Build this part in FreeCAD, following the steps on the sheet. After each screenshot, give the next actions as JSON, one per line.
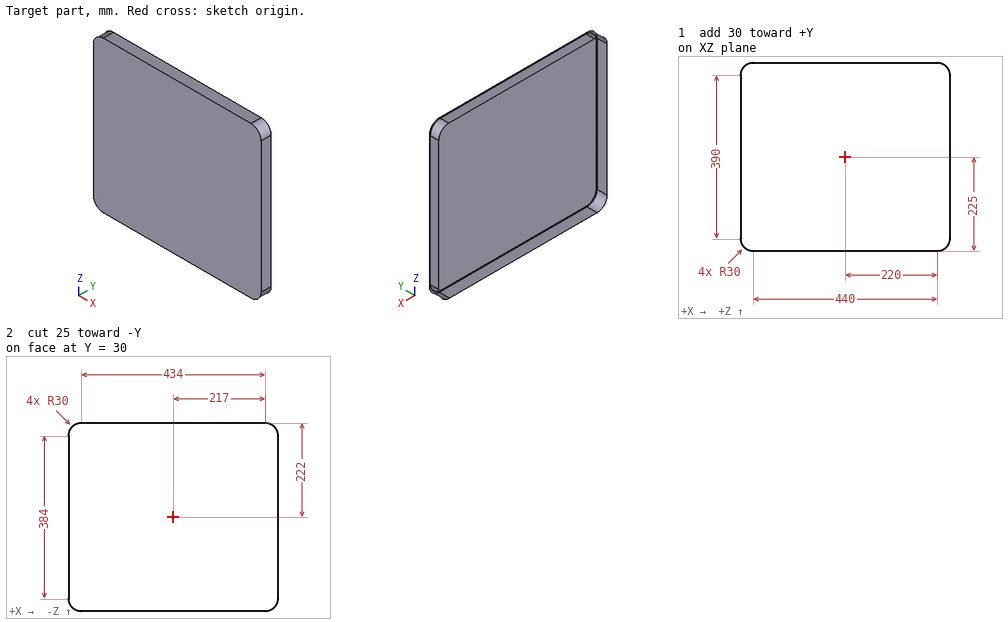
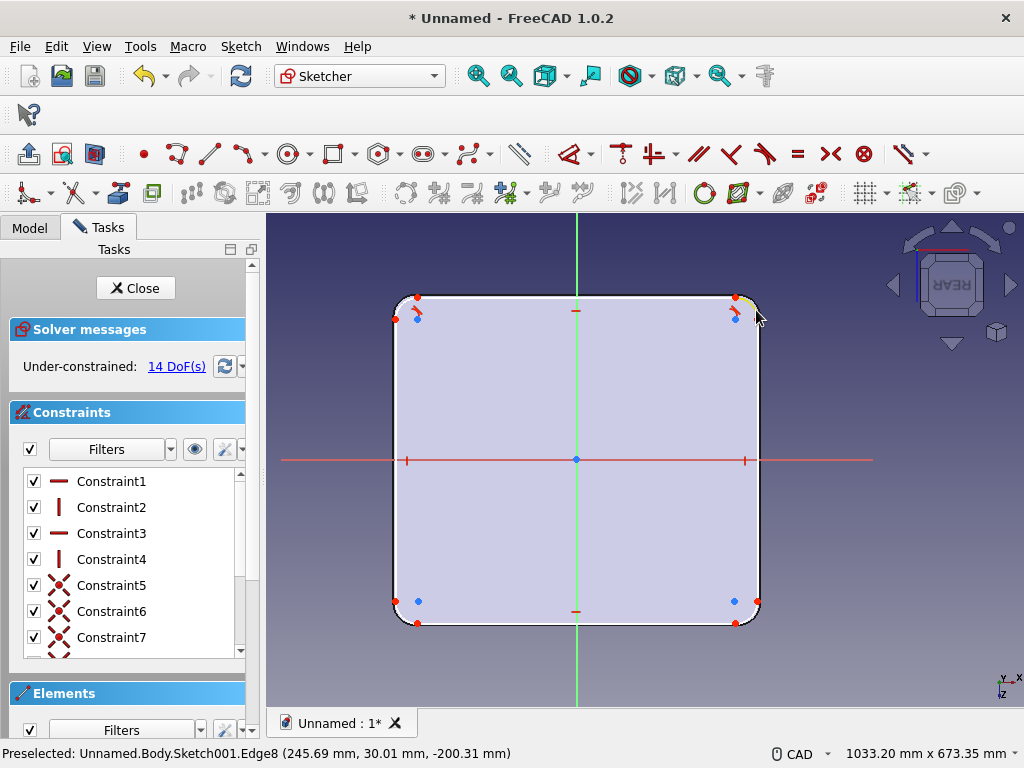
{"action": "left_click", "coordinate": [396, 405]}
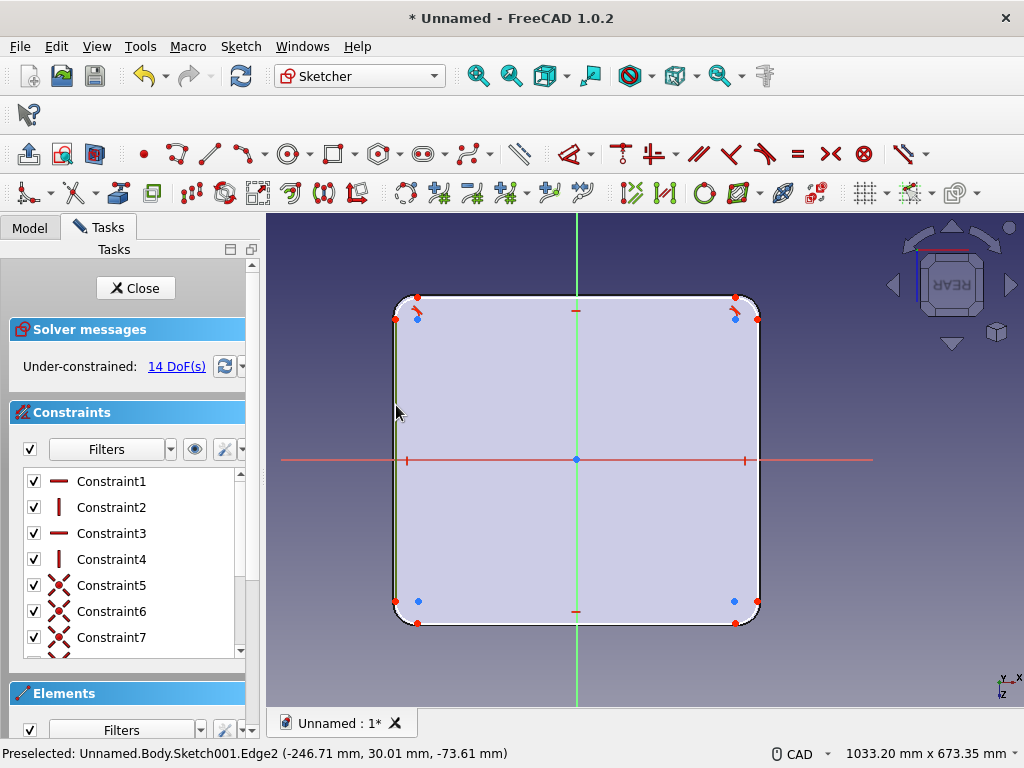
{"action": "scroll", "coordinate": [408, 300], "scroll_direction": "up", "scroll_amount": 2}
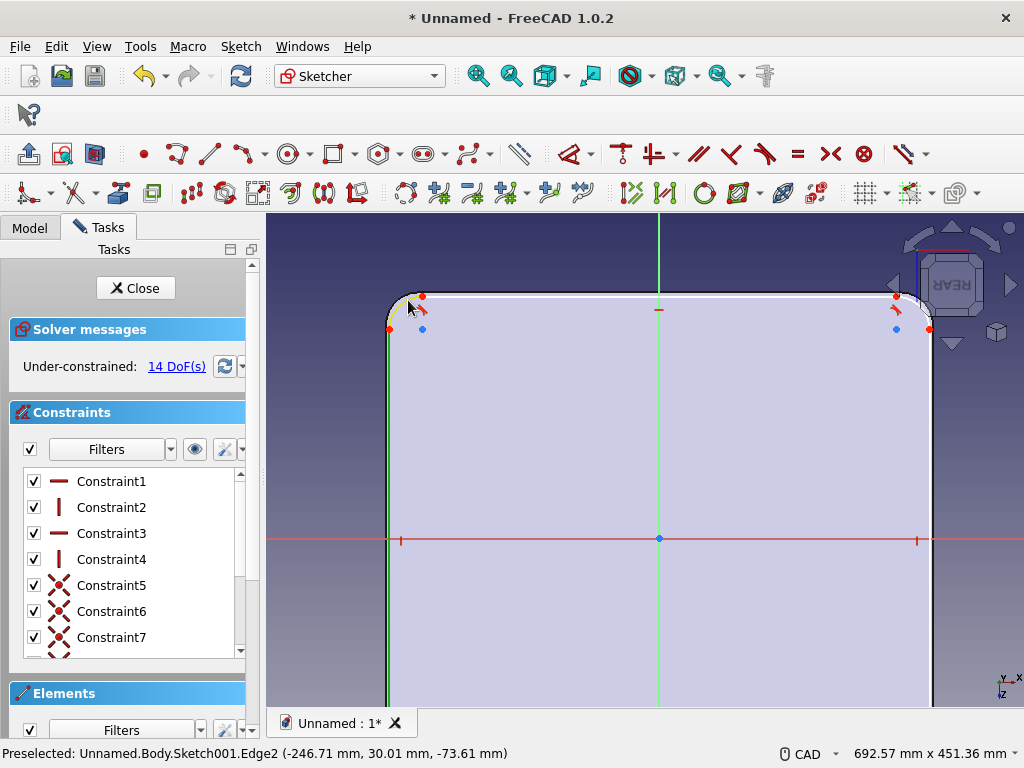
{"action": "left_click", "coordinate": [407, 301]}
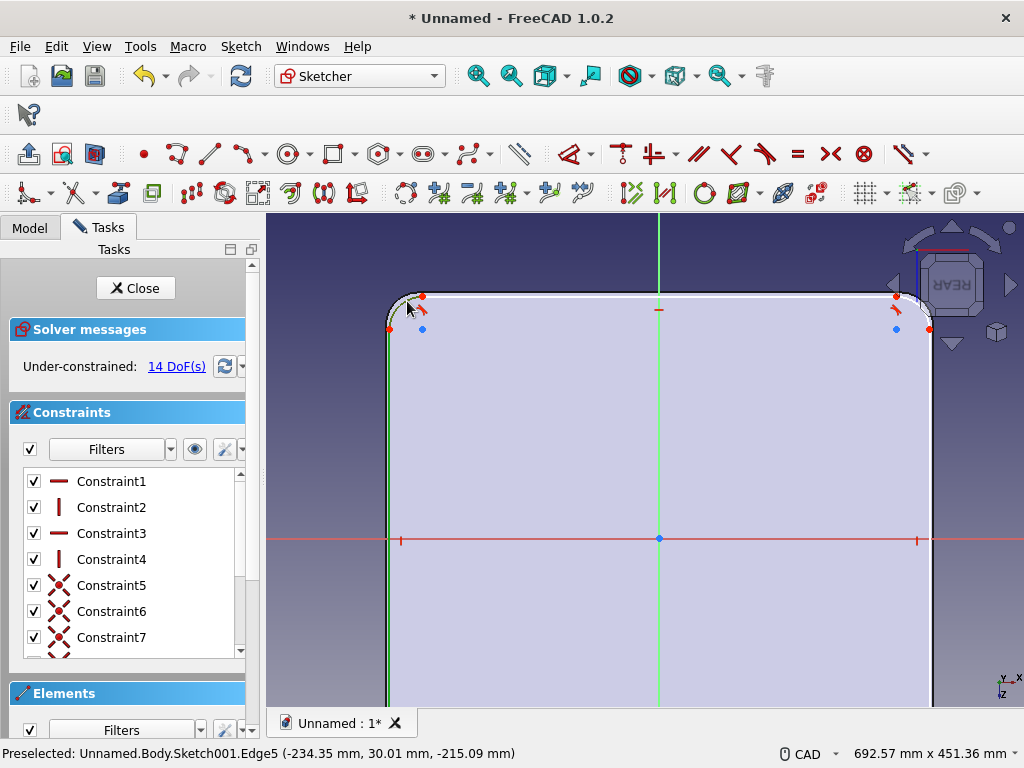
{"action": "left_click", "coordinate": [765, 154]}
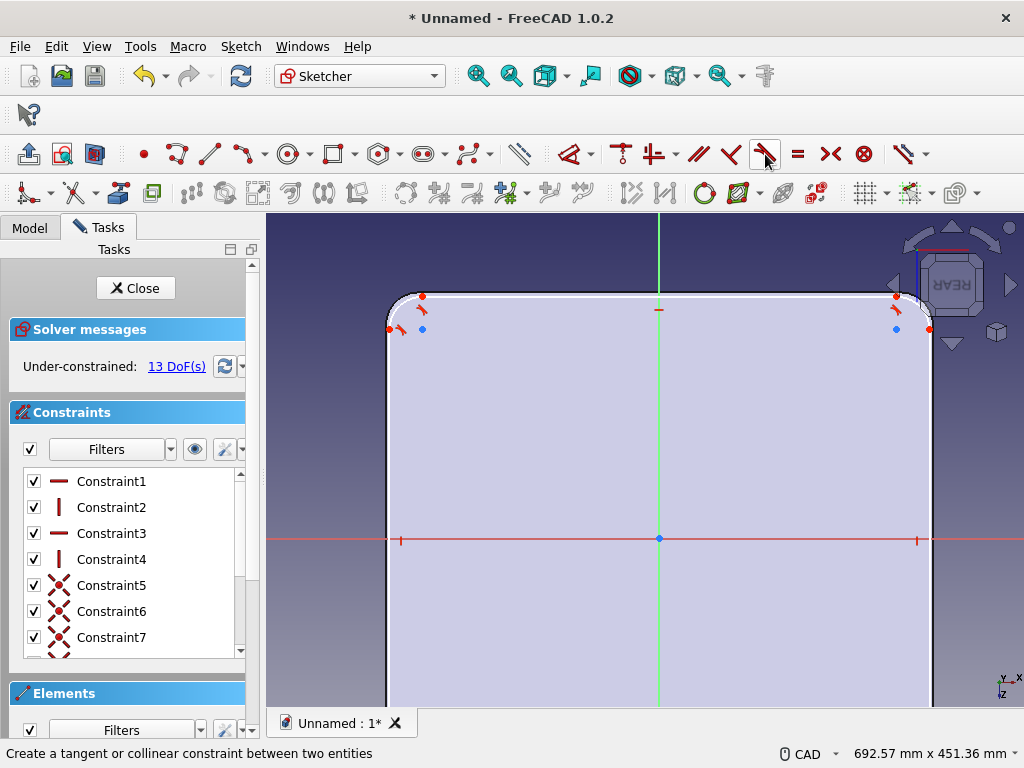
{"action": "left_click", "coordinate": [389, 456]}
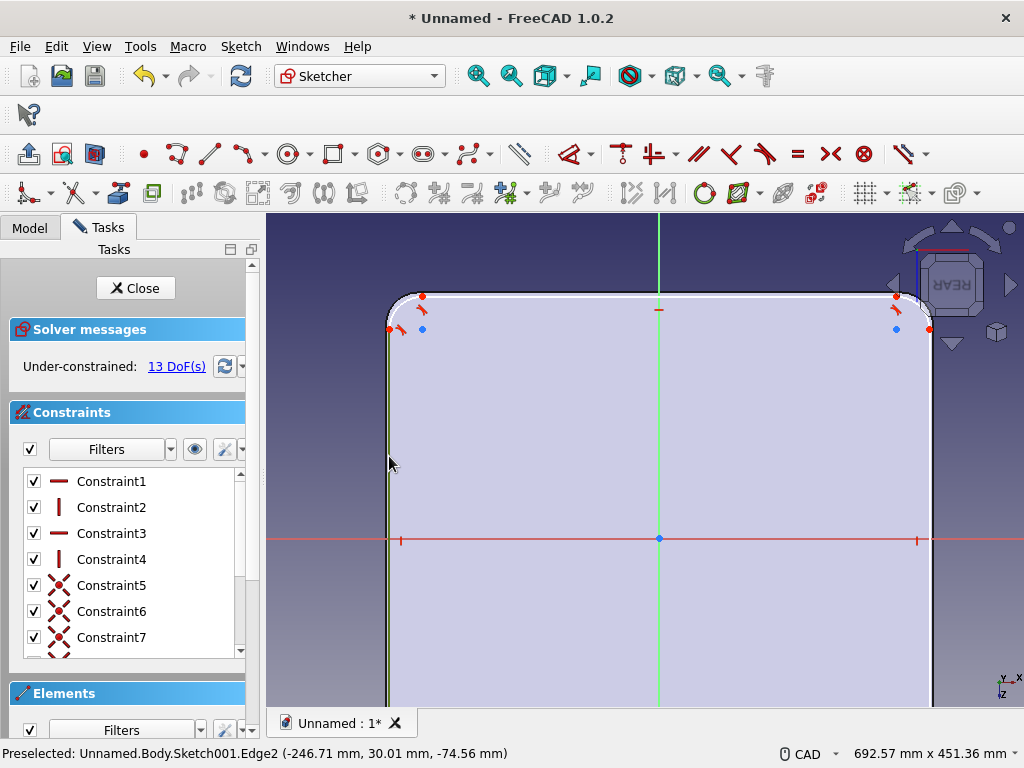
{"action": "scroll", "coordinate": [408, 300], "scroll_direction": "down", "scroll_amount": 2}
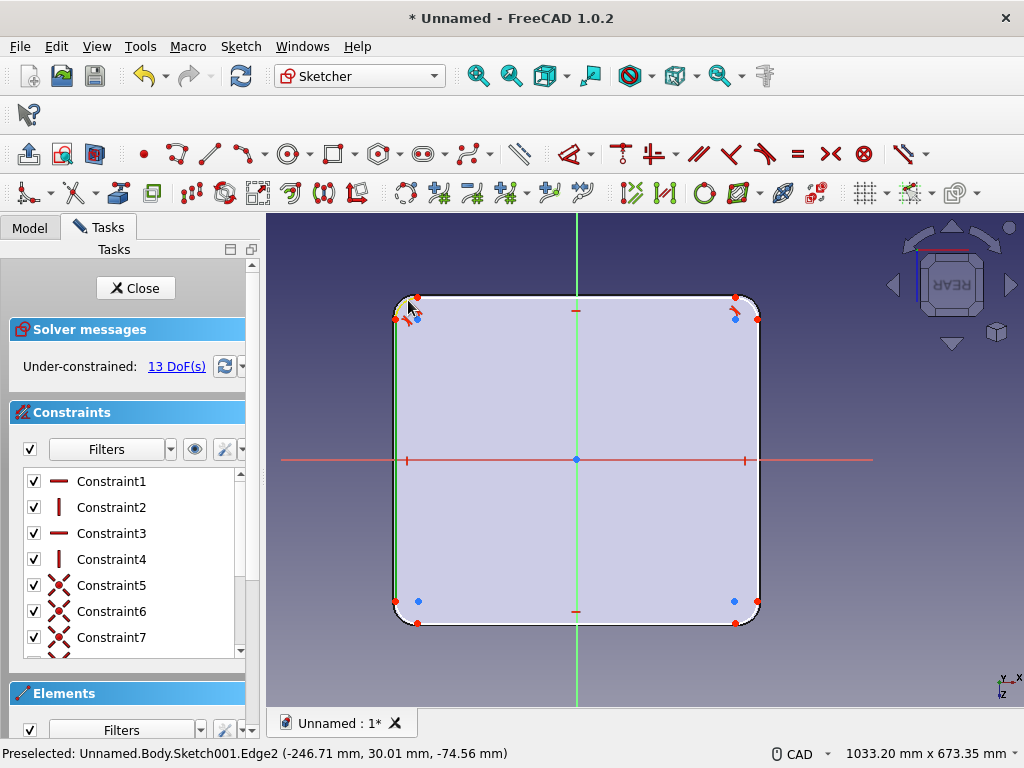
{"action": "scroll", "coordinate": [398, 612], "scroll_direction": "up", "scroll_amount": 2}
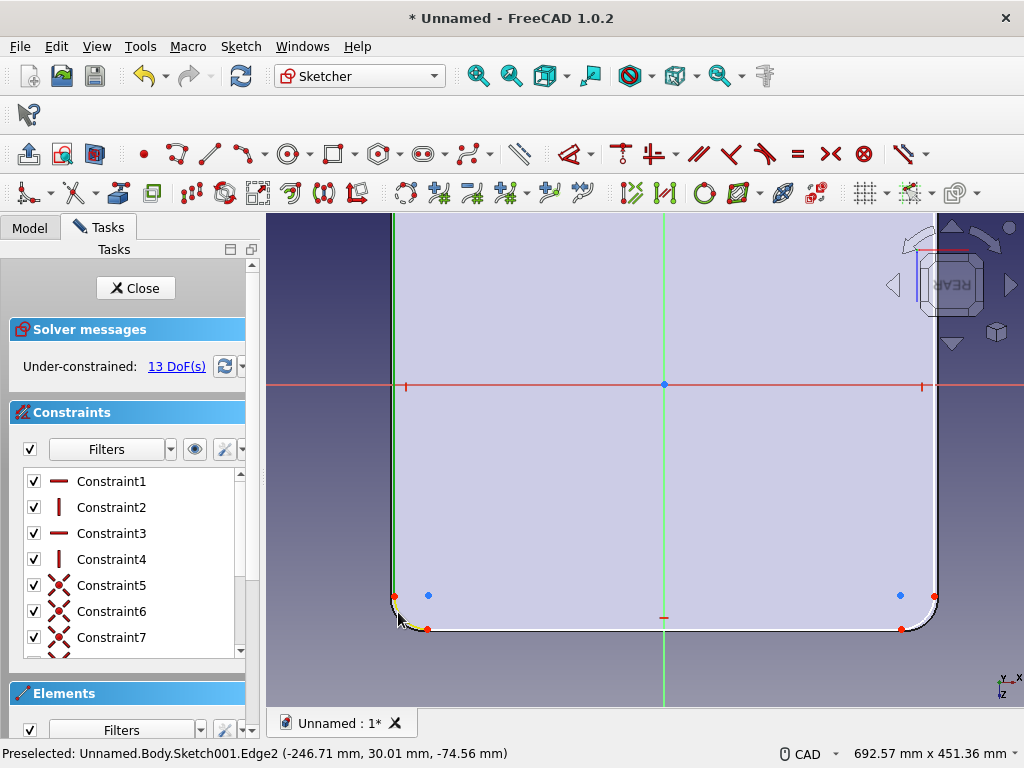
{"action": "left_click", "coordinate": [398, 611]}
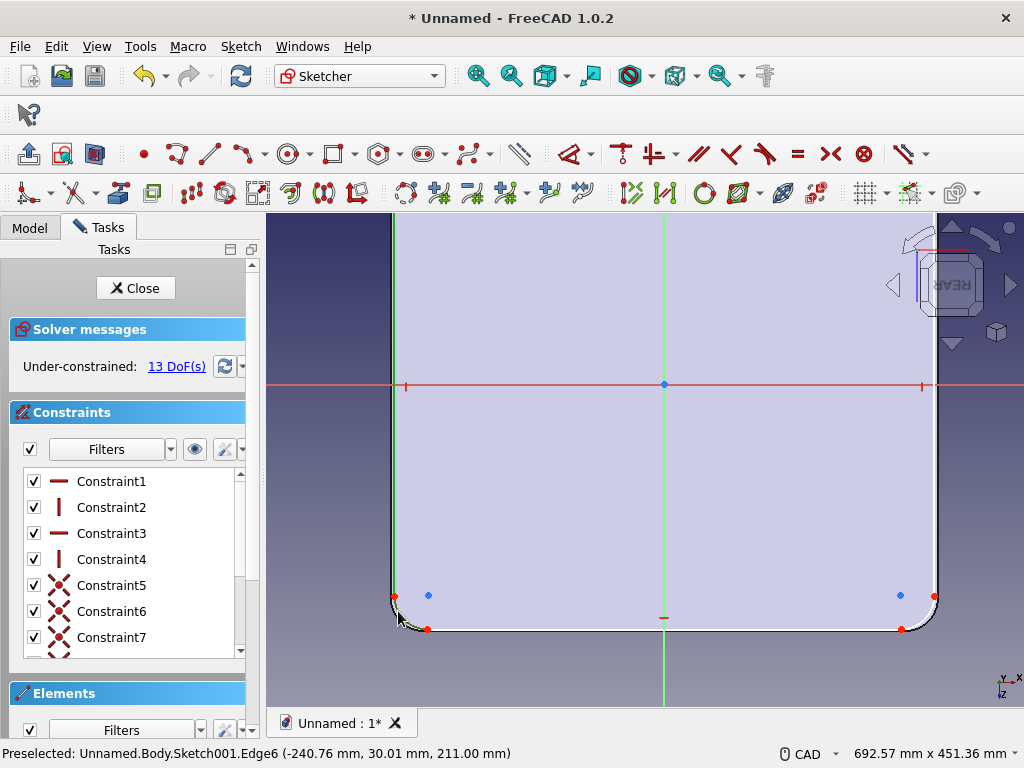
{"action": "left_click", "coordinate": [765, 154]}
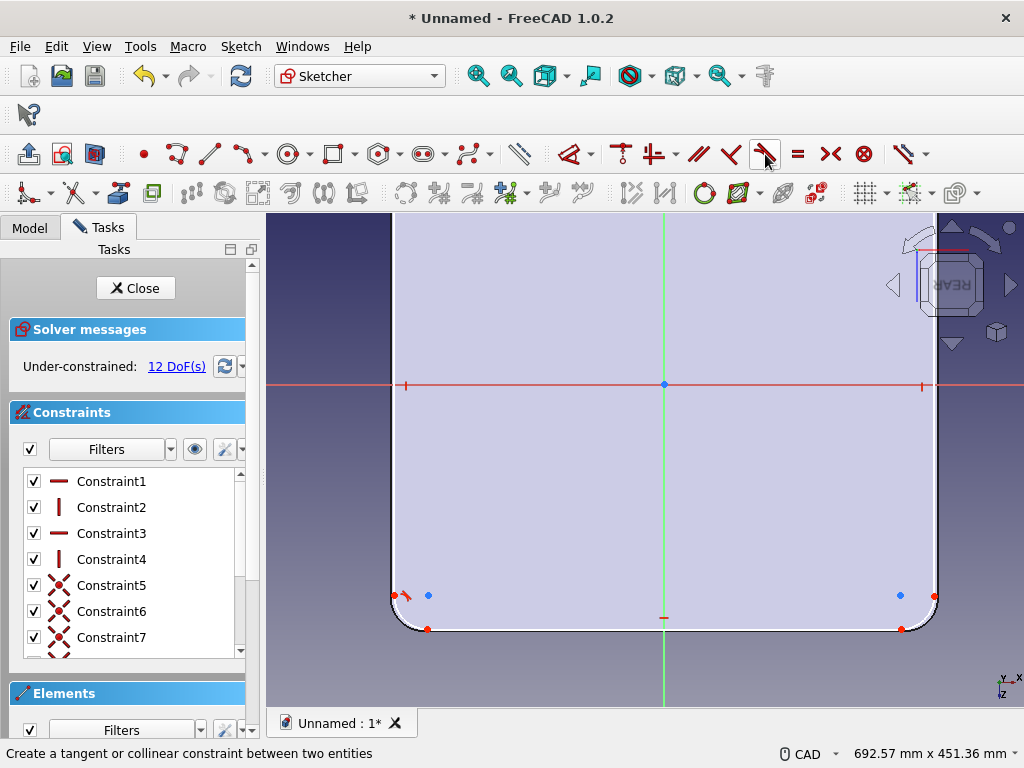
{"action": "left_click", "coordinate": [570, 630]}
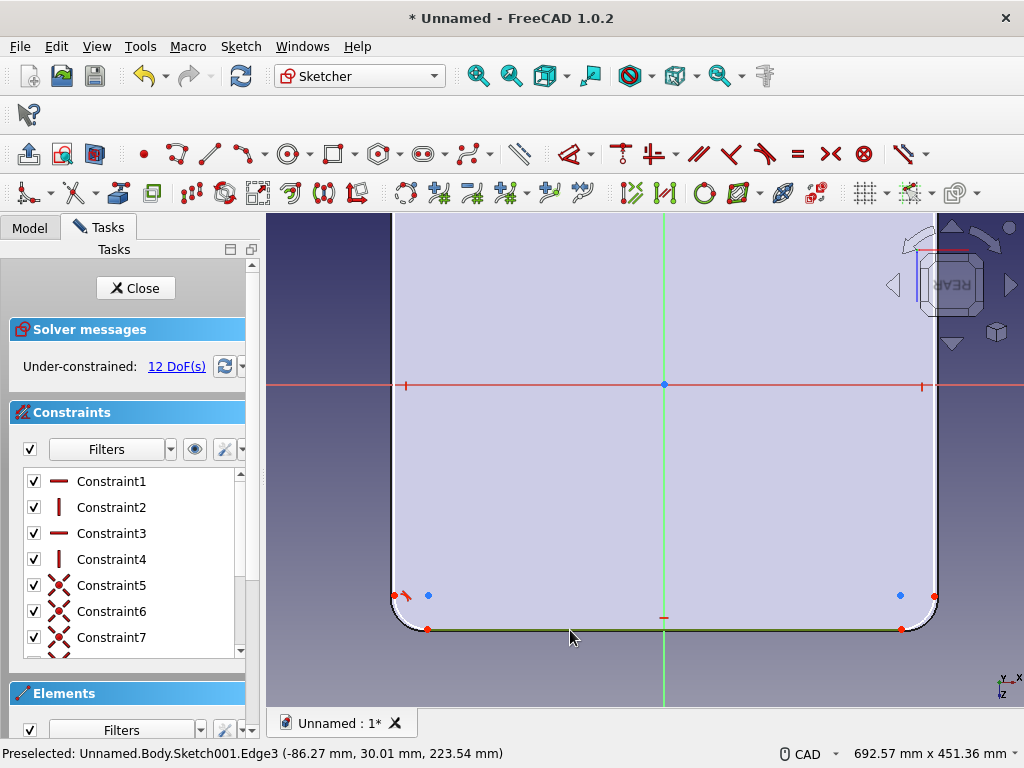
{"action": "left_click", "coordinate": [398, 611]}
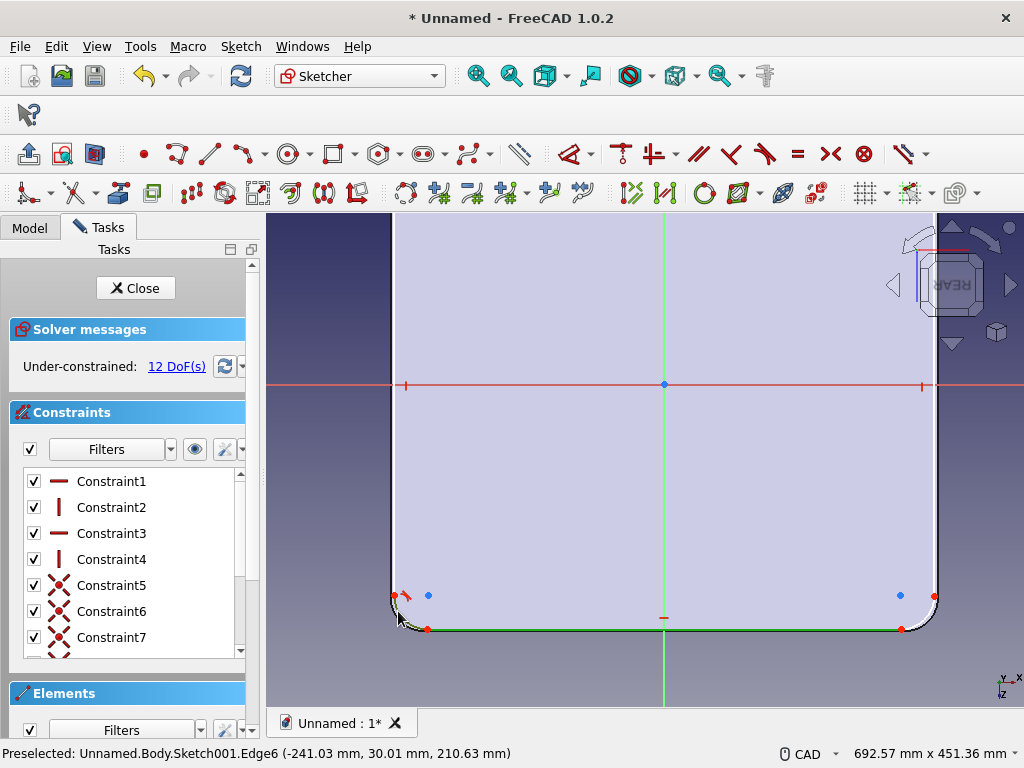
{"action": "left_click", "coordinate": [765, 154]}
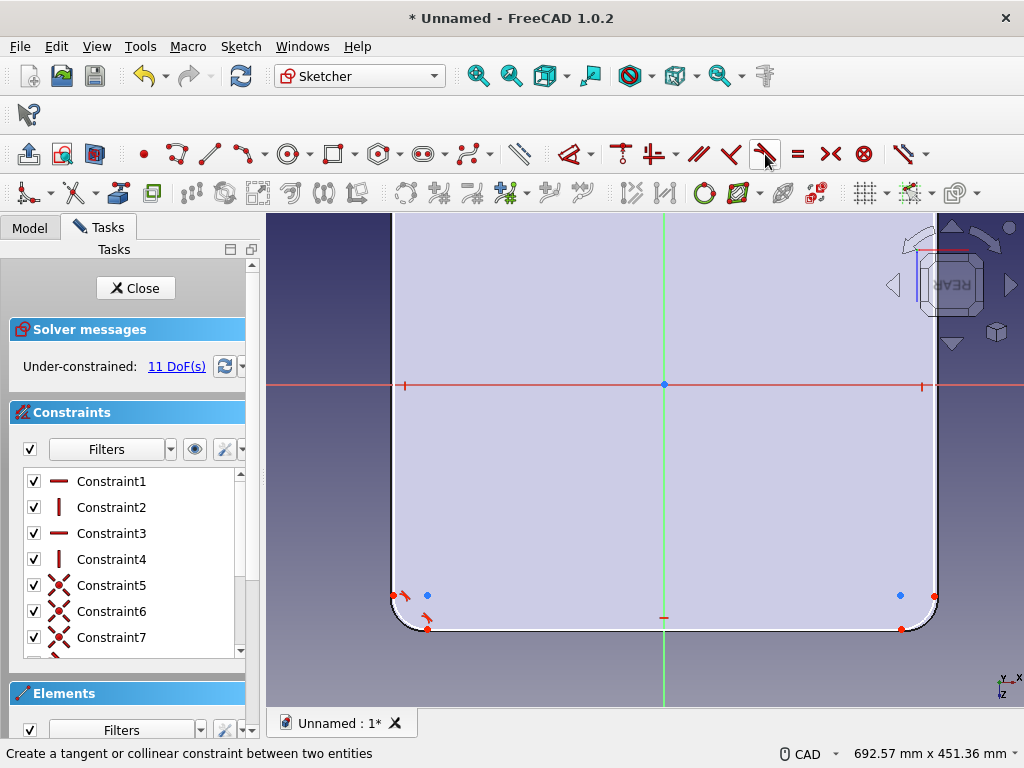
{"action": "left_click", "coordinate": [570, 630]}